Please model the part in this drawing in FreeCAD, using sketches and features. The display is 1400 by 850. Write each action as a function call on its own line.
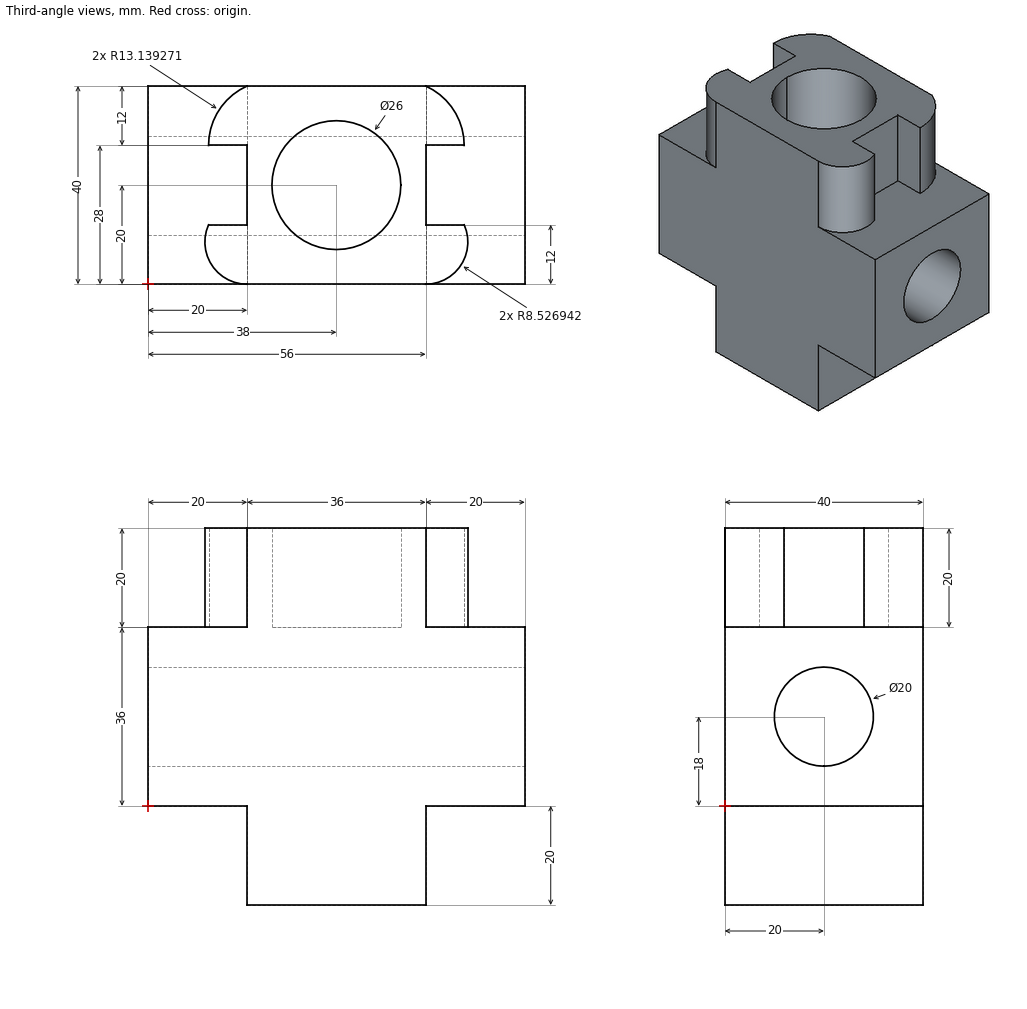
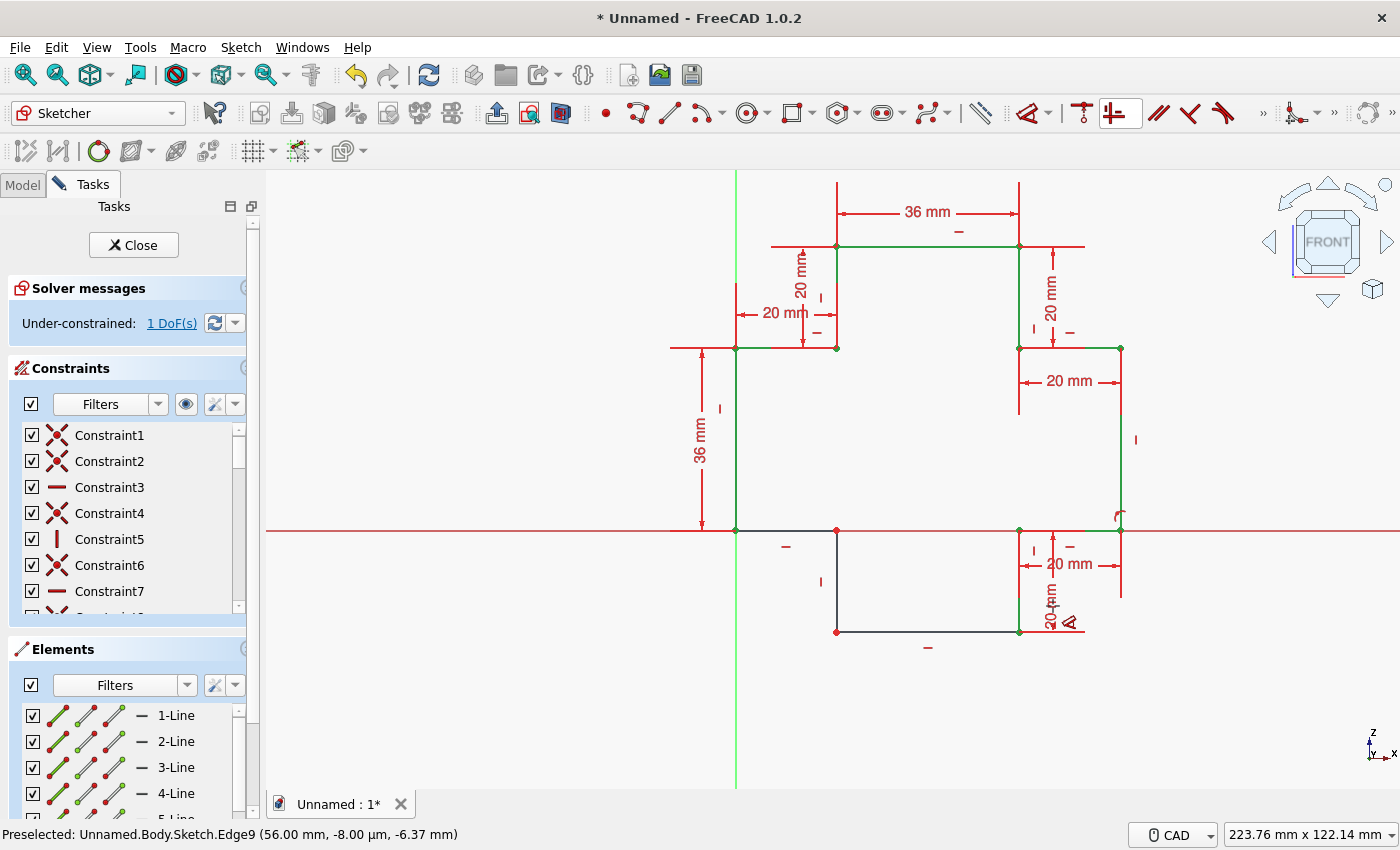
click(965, 632)
click(928, 666)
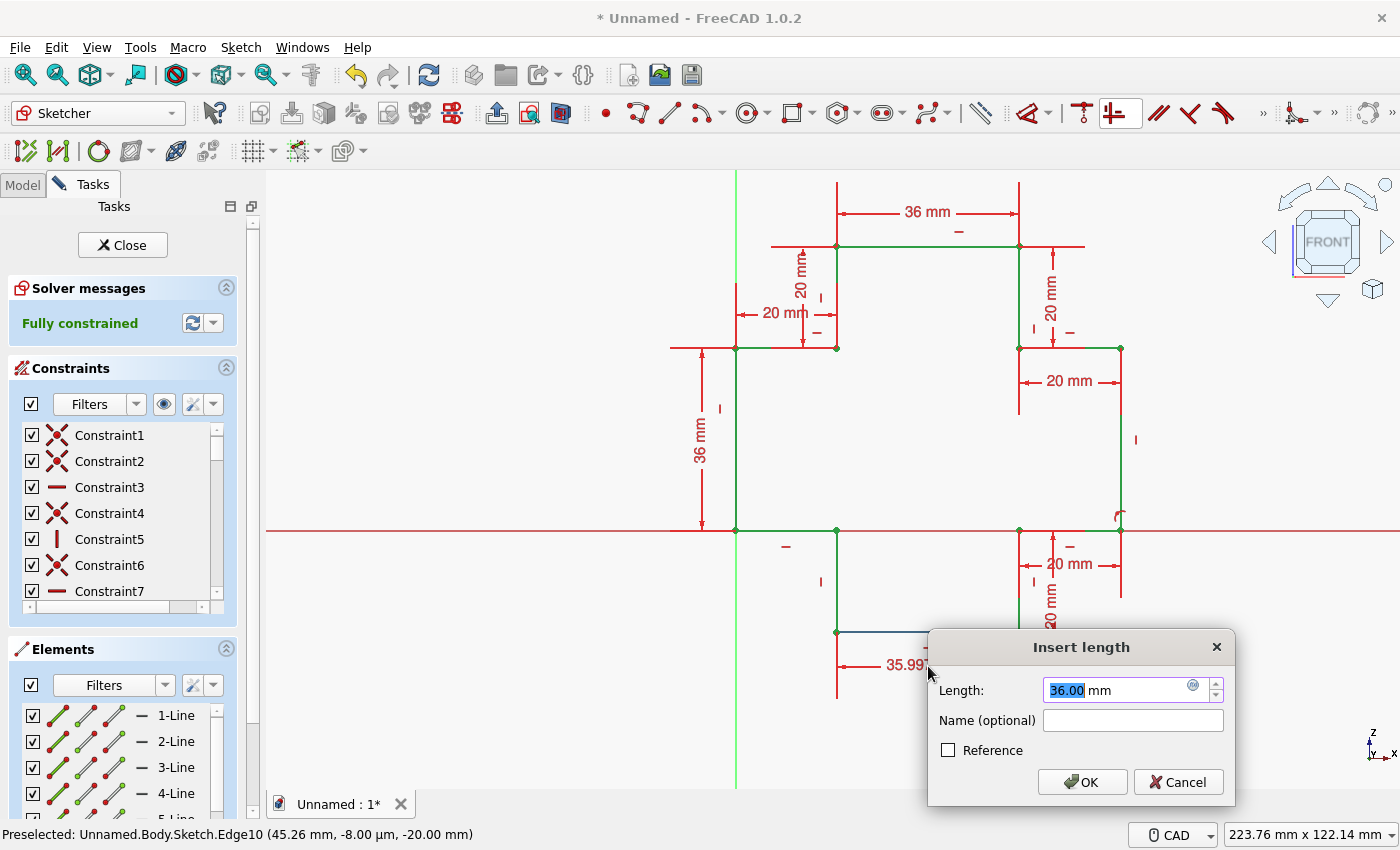
text(36)
key(Return)
key(Escape)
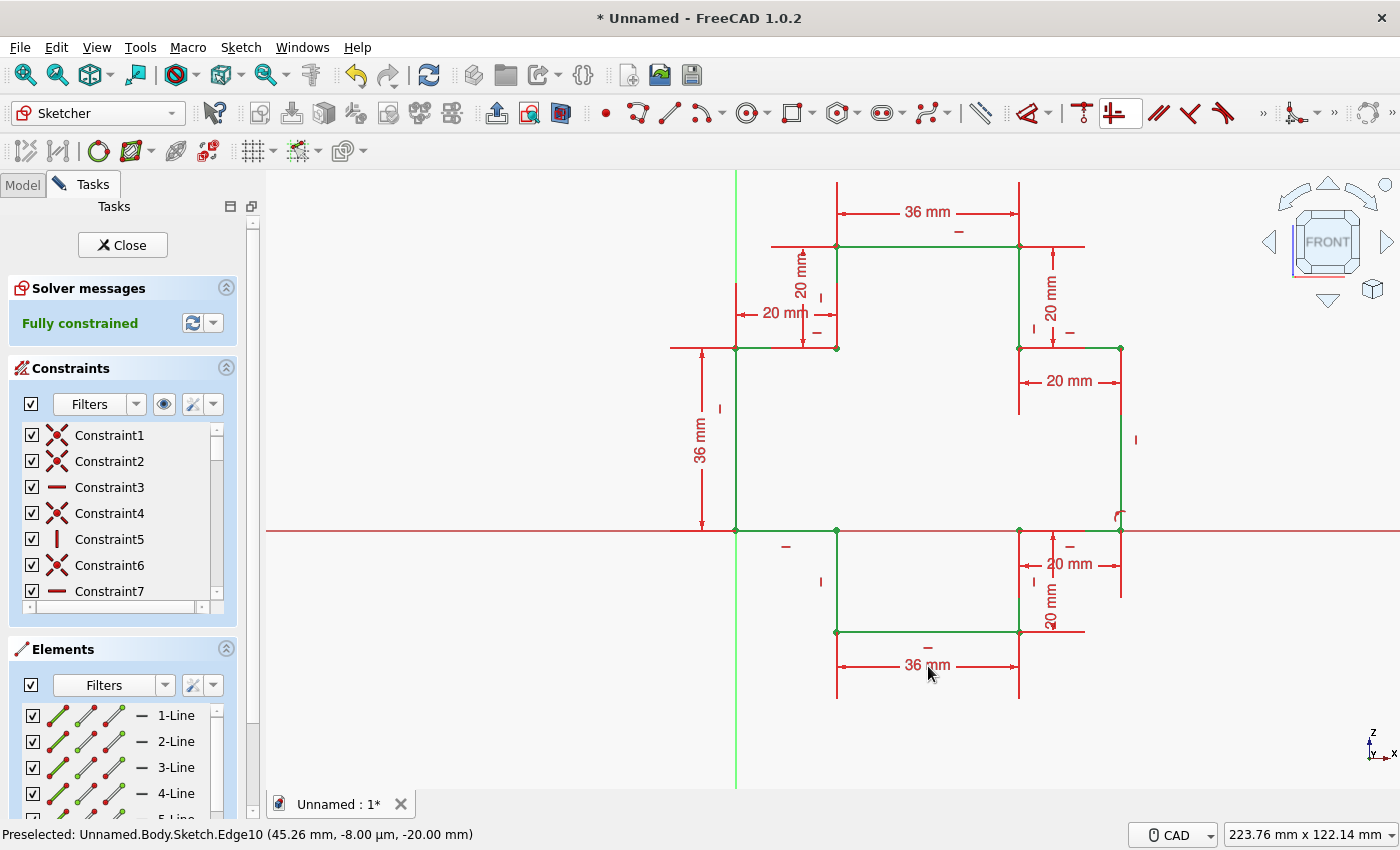
click(123, 245)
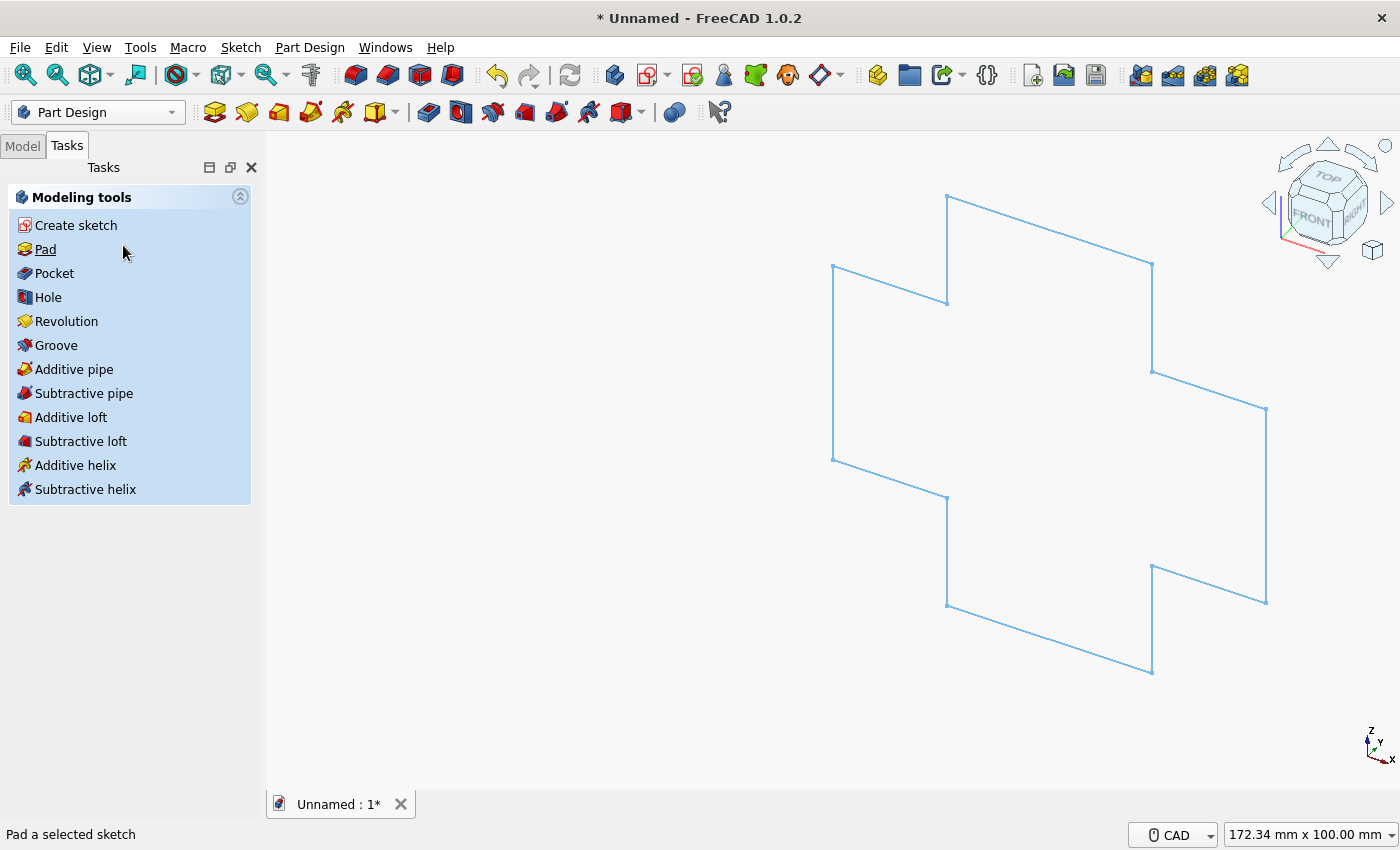
click(216, 112)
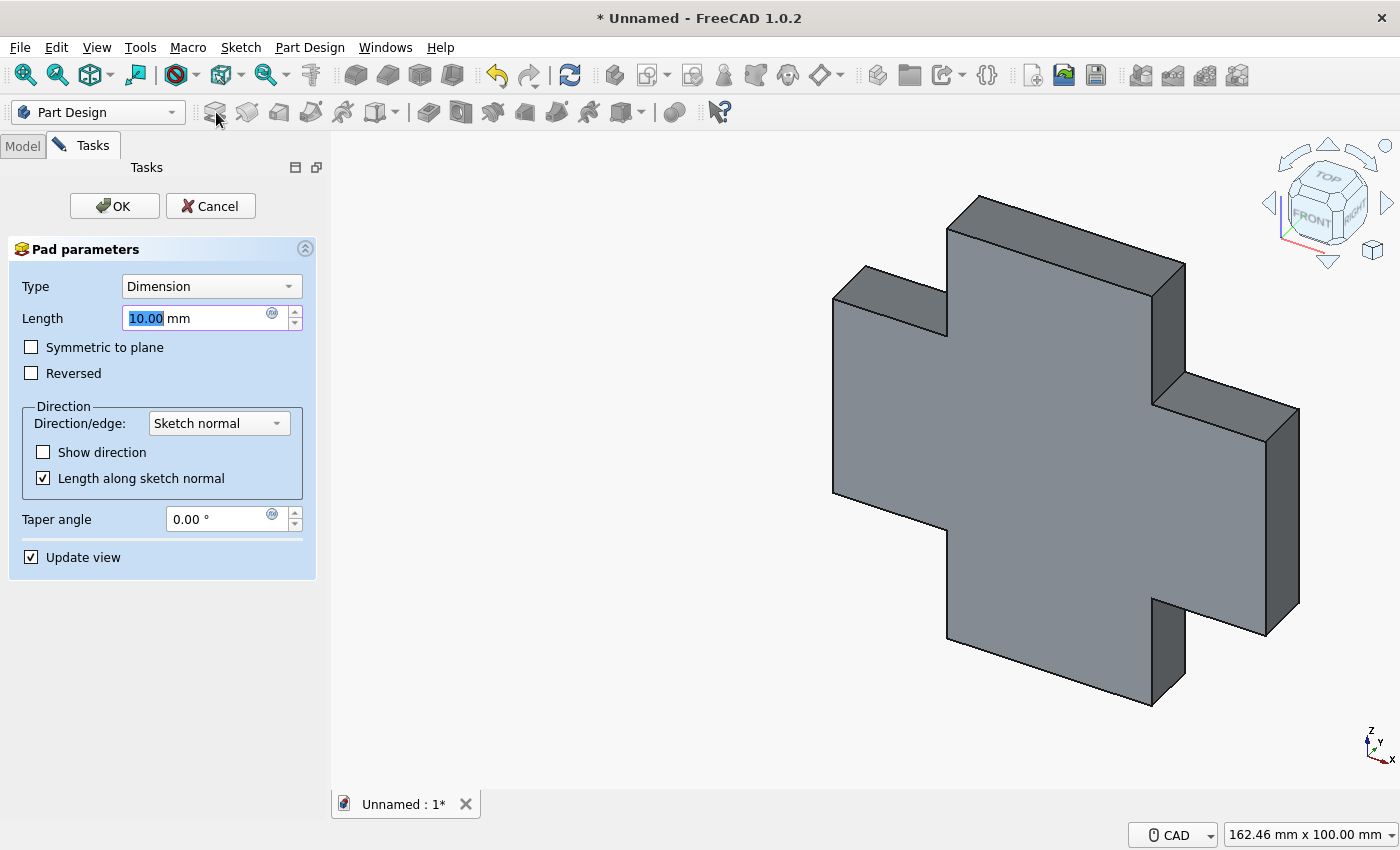
text(40)
key(Tab)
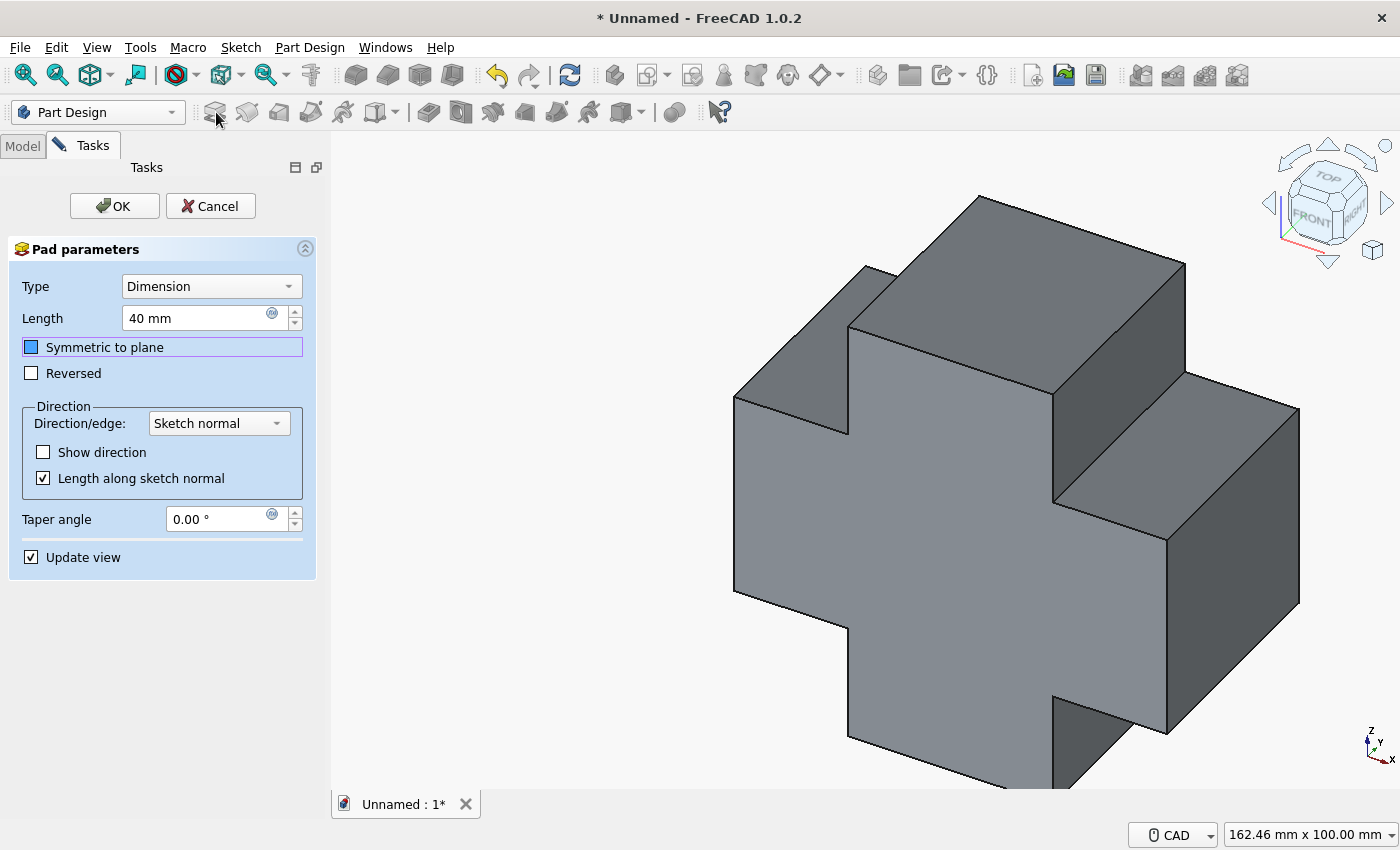
click(30, 373)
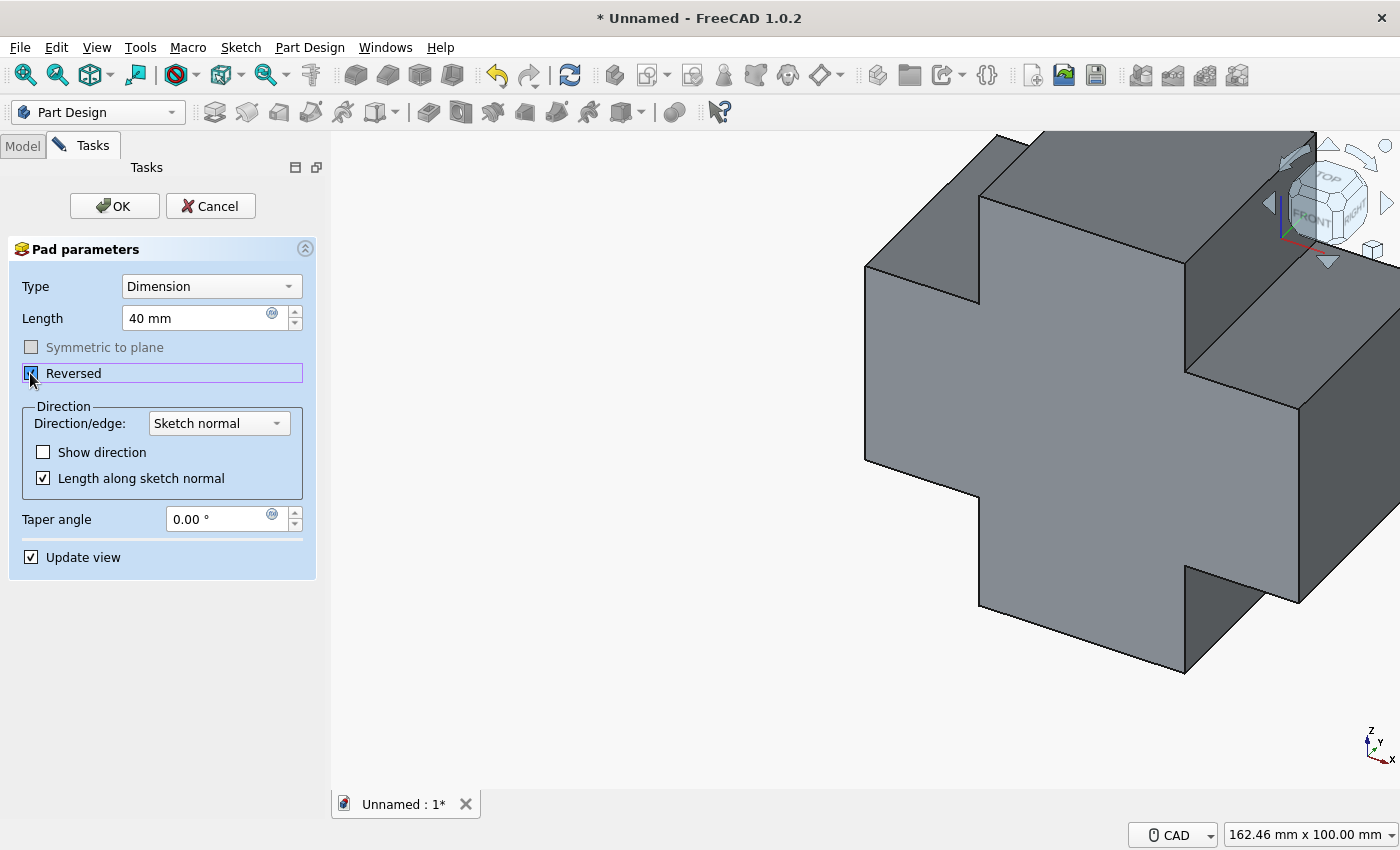
click(115, 206)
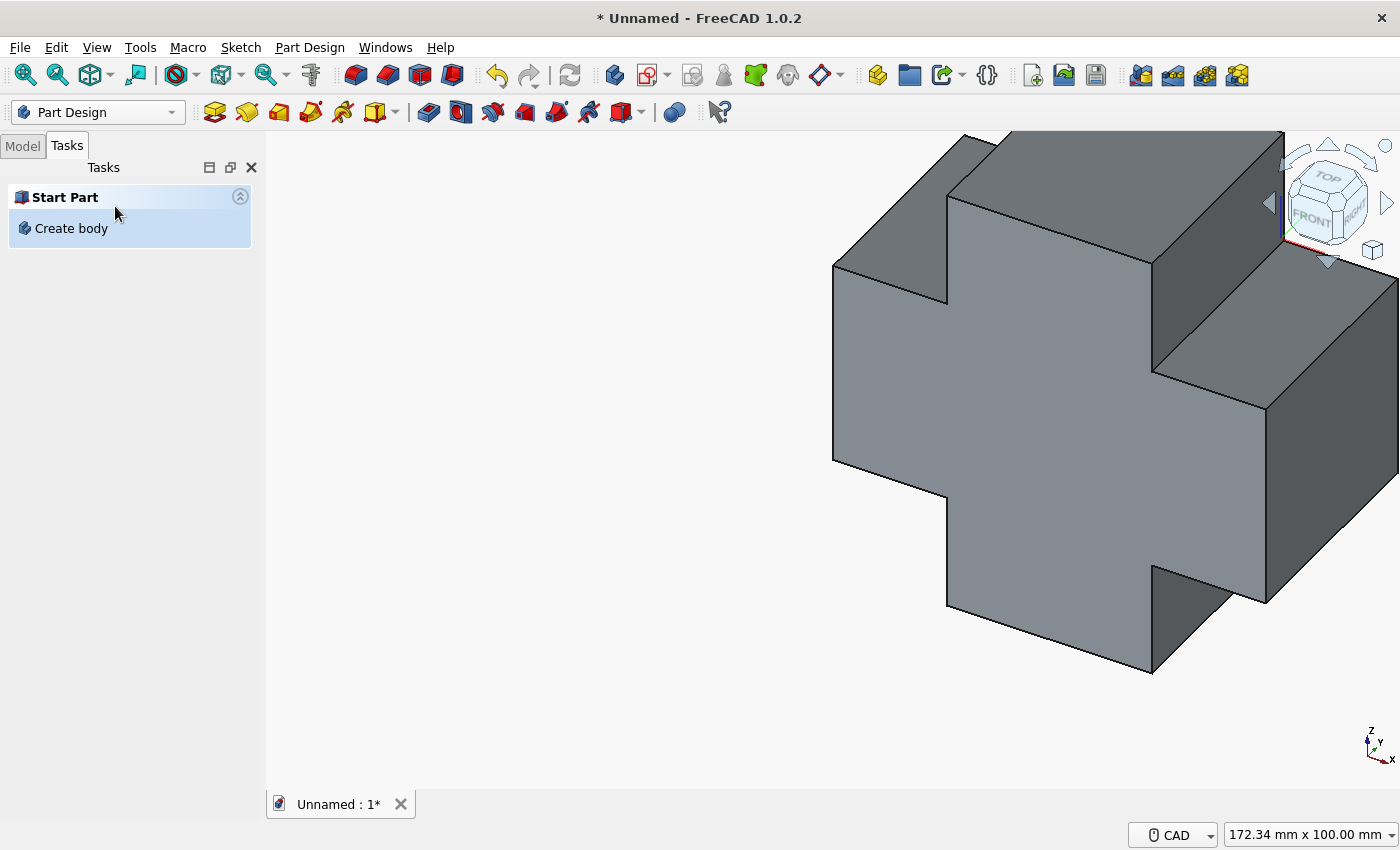
click(26, 76)